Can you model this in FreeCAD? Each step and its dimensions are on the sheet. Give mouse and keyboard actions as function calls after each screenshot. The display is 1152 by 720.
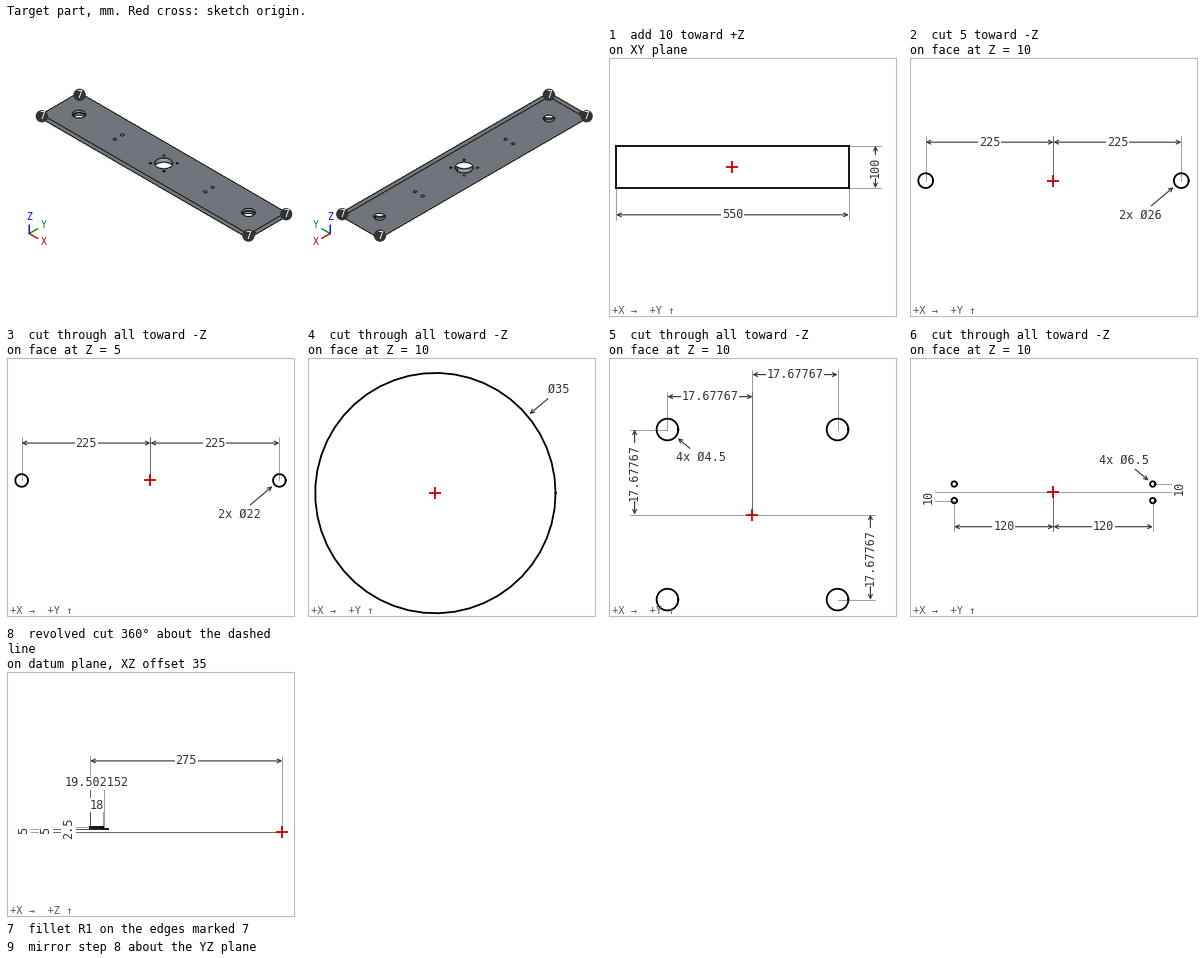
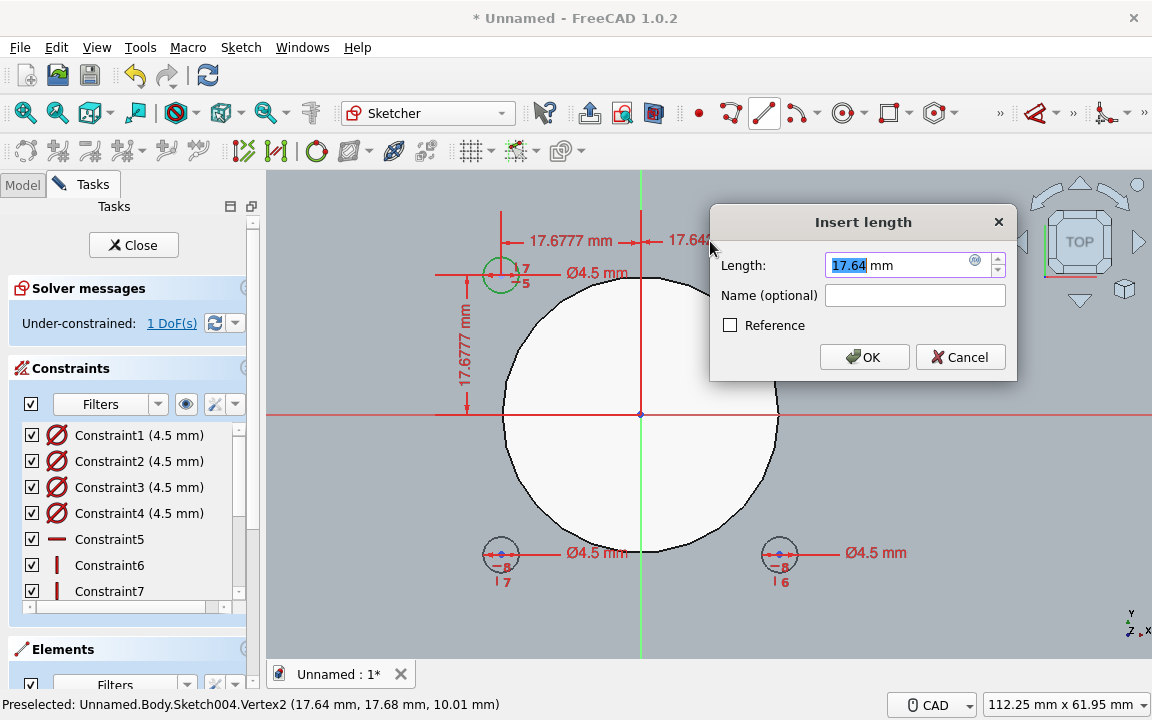
text(17.67767)
key(Return)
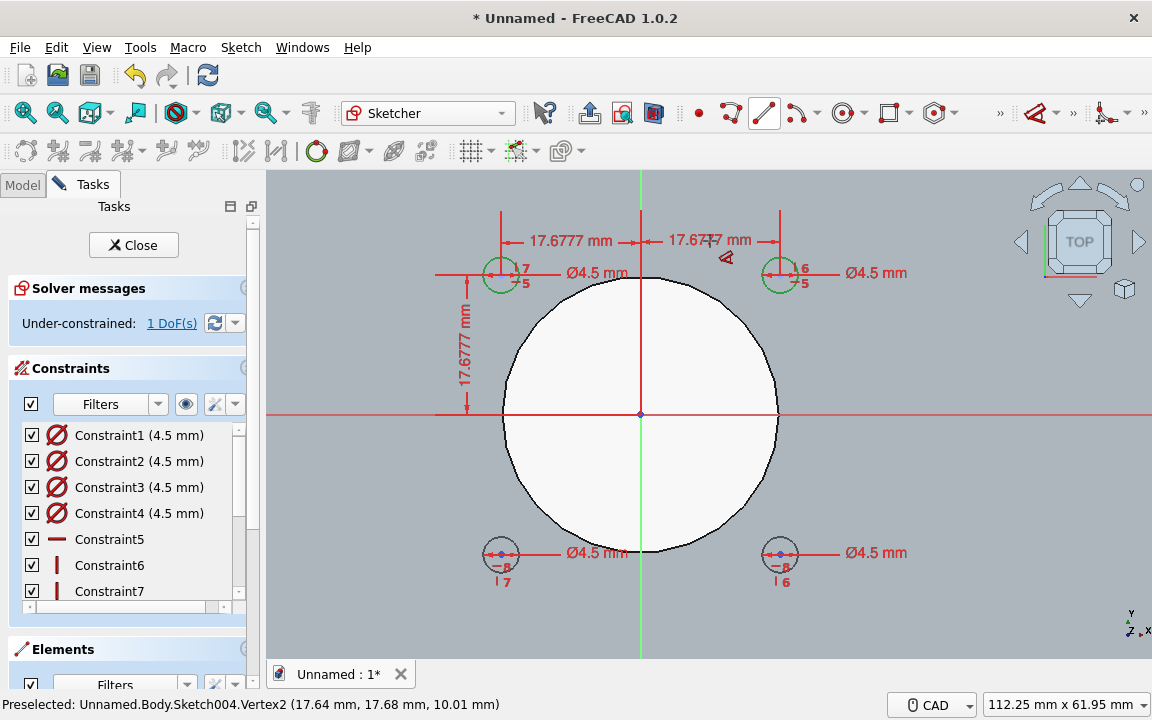
click(780, 555)
click(814, 485)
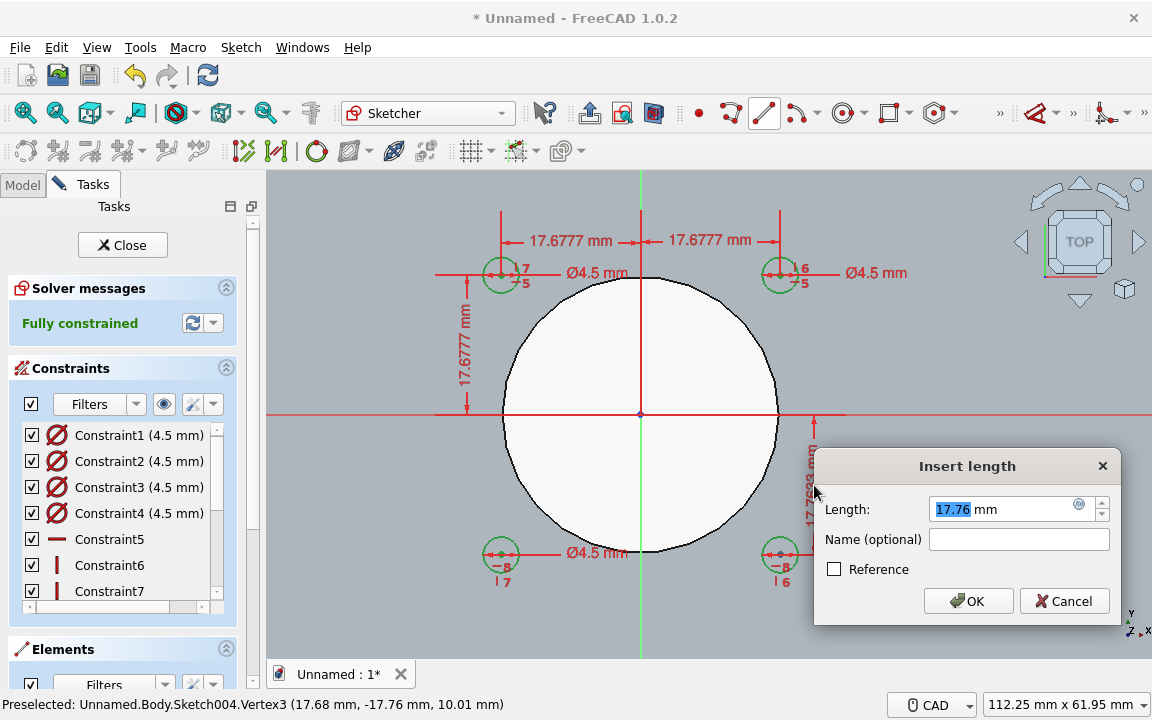
text(17.67767)
key(Return)
key(Escape)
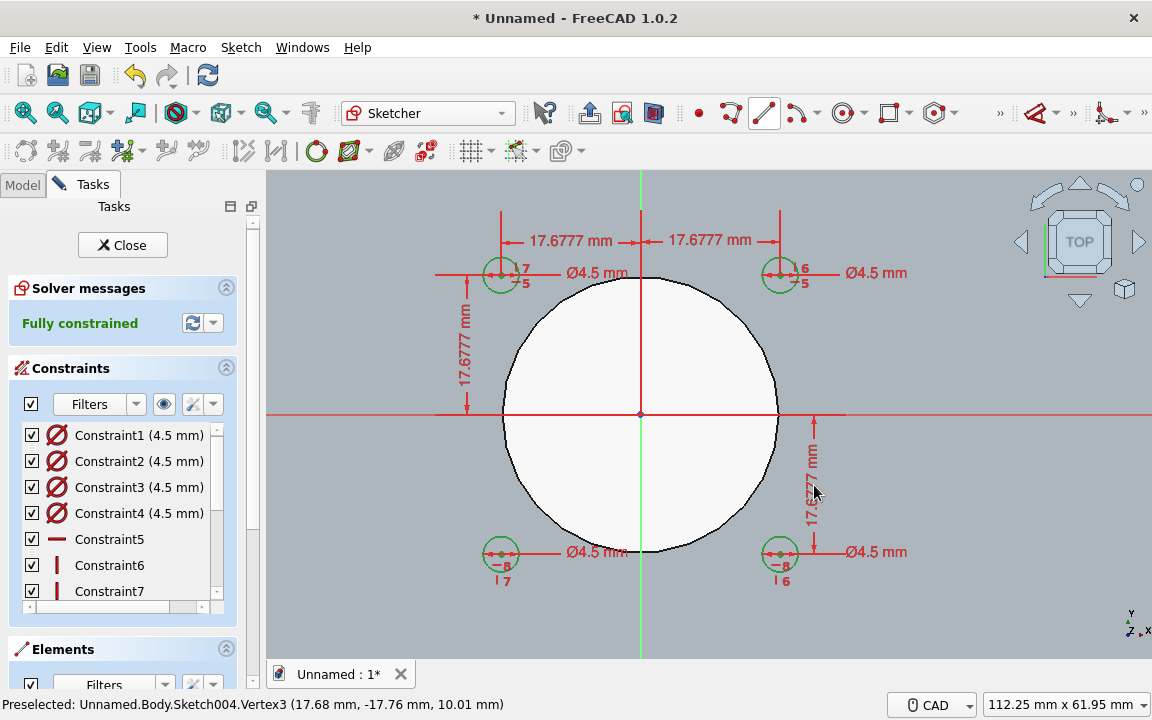
click(123, 245)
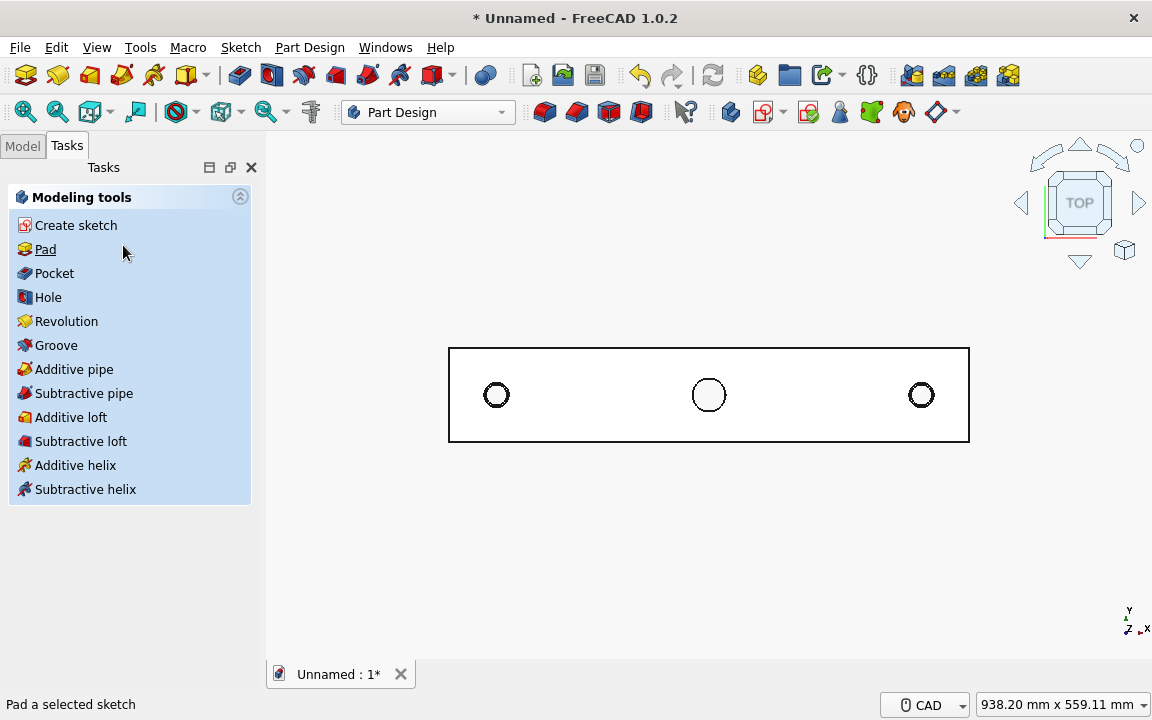
click(240, 76)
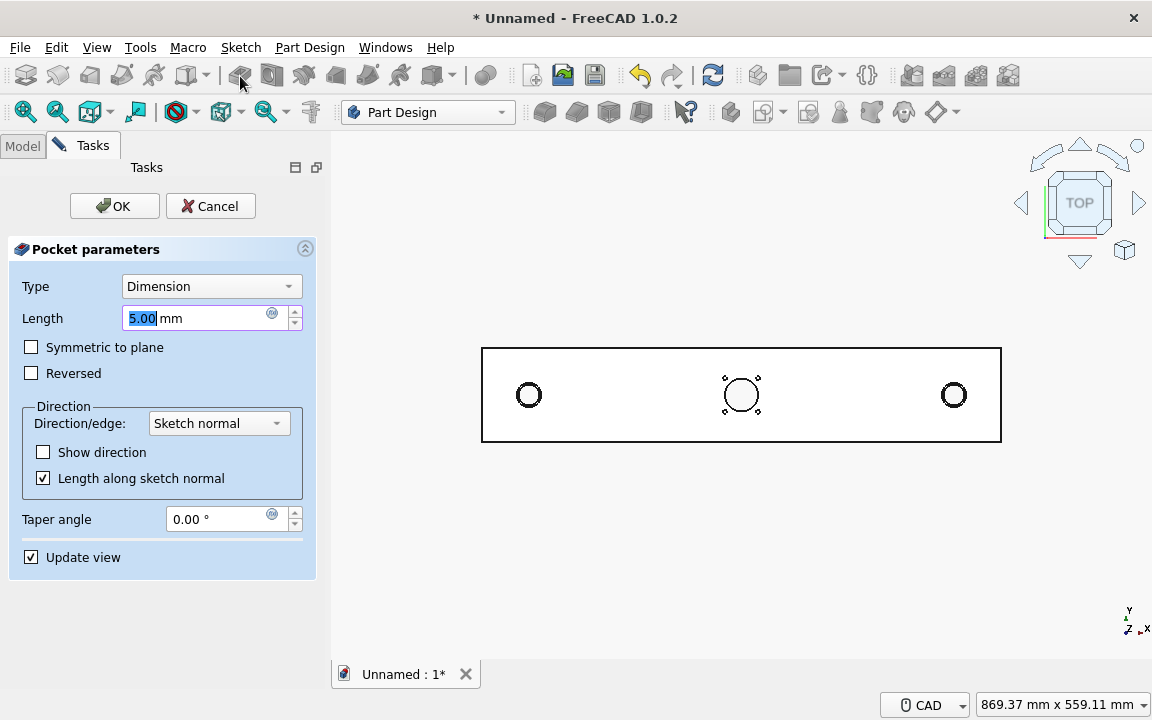
click(212, 286)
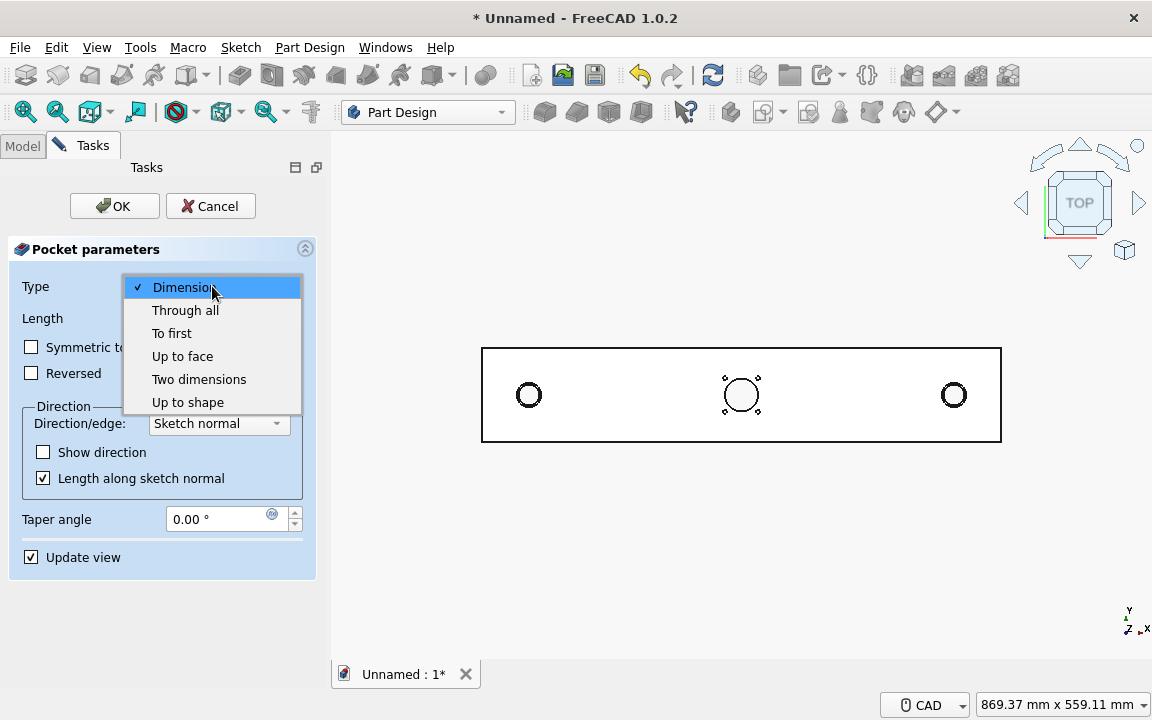
click(212, 310)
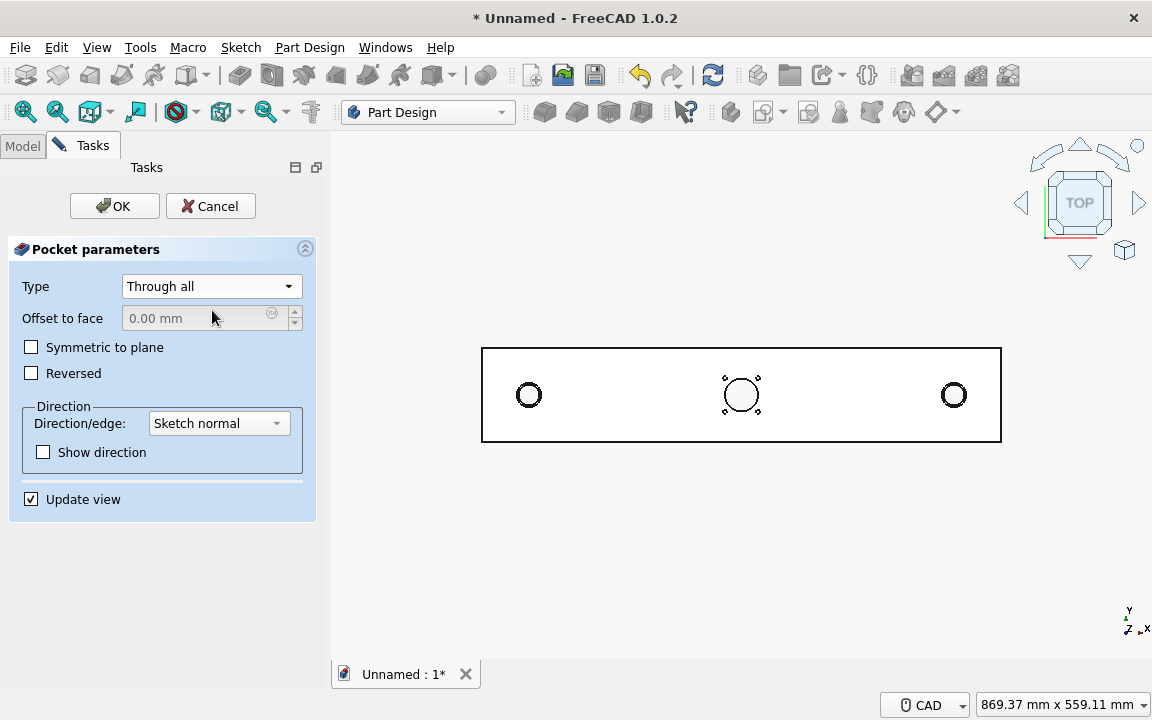
click(115, 206)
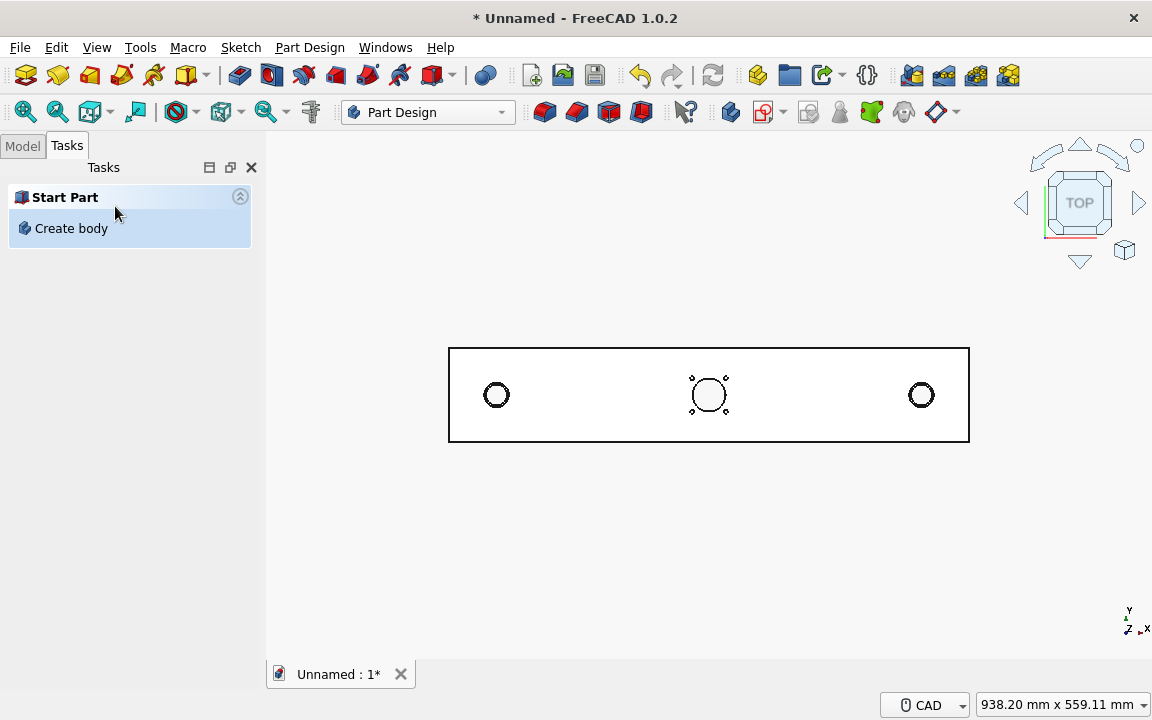
click(857, 394)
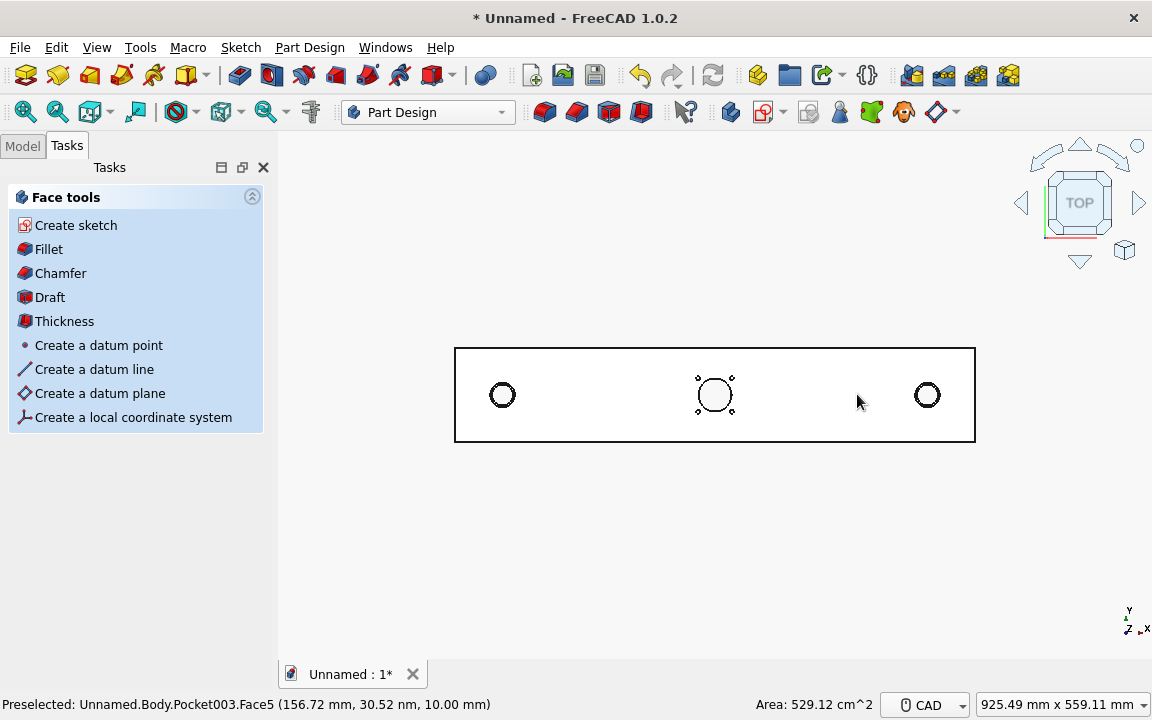
click(764, 112)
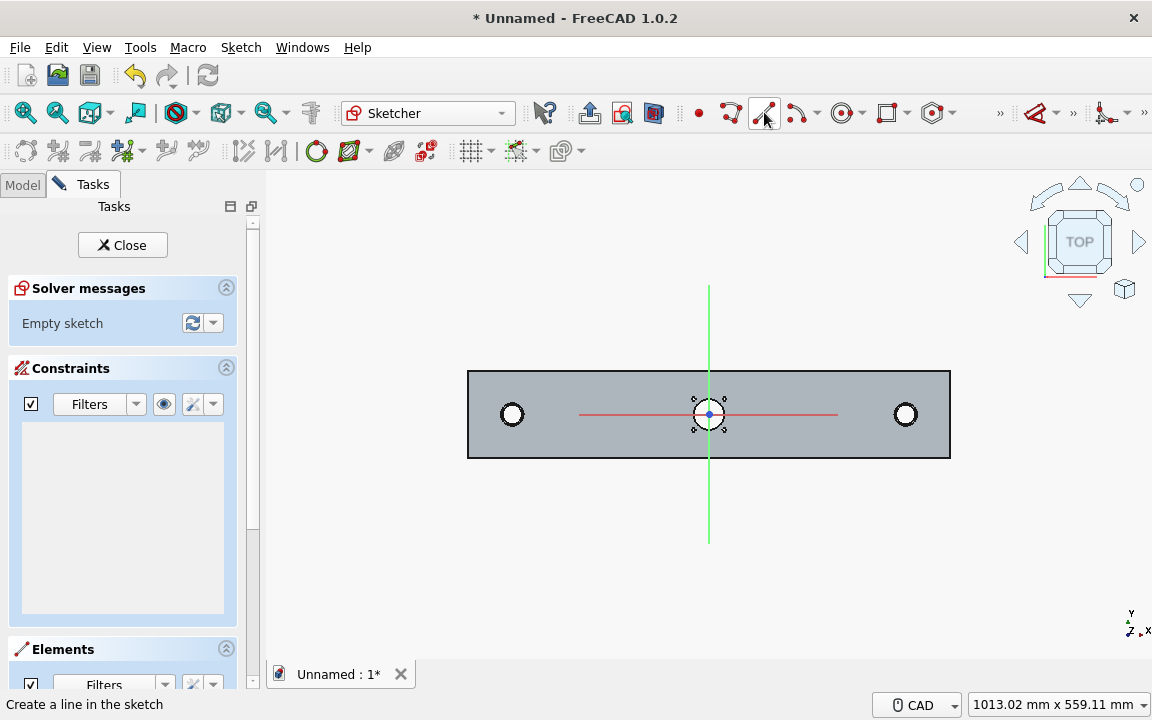
scroll(765, 415, up, 4)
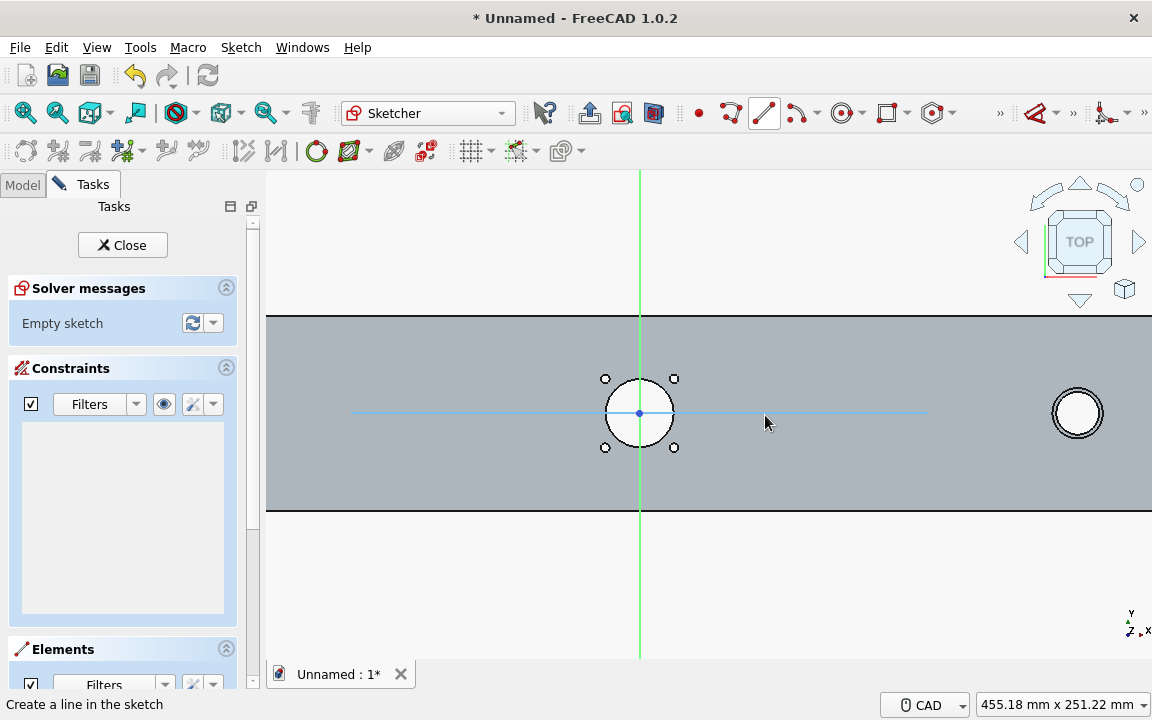
click(842, 114)